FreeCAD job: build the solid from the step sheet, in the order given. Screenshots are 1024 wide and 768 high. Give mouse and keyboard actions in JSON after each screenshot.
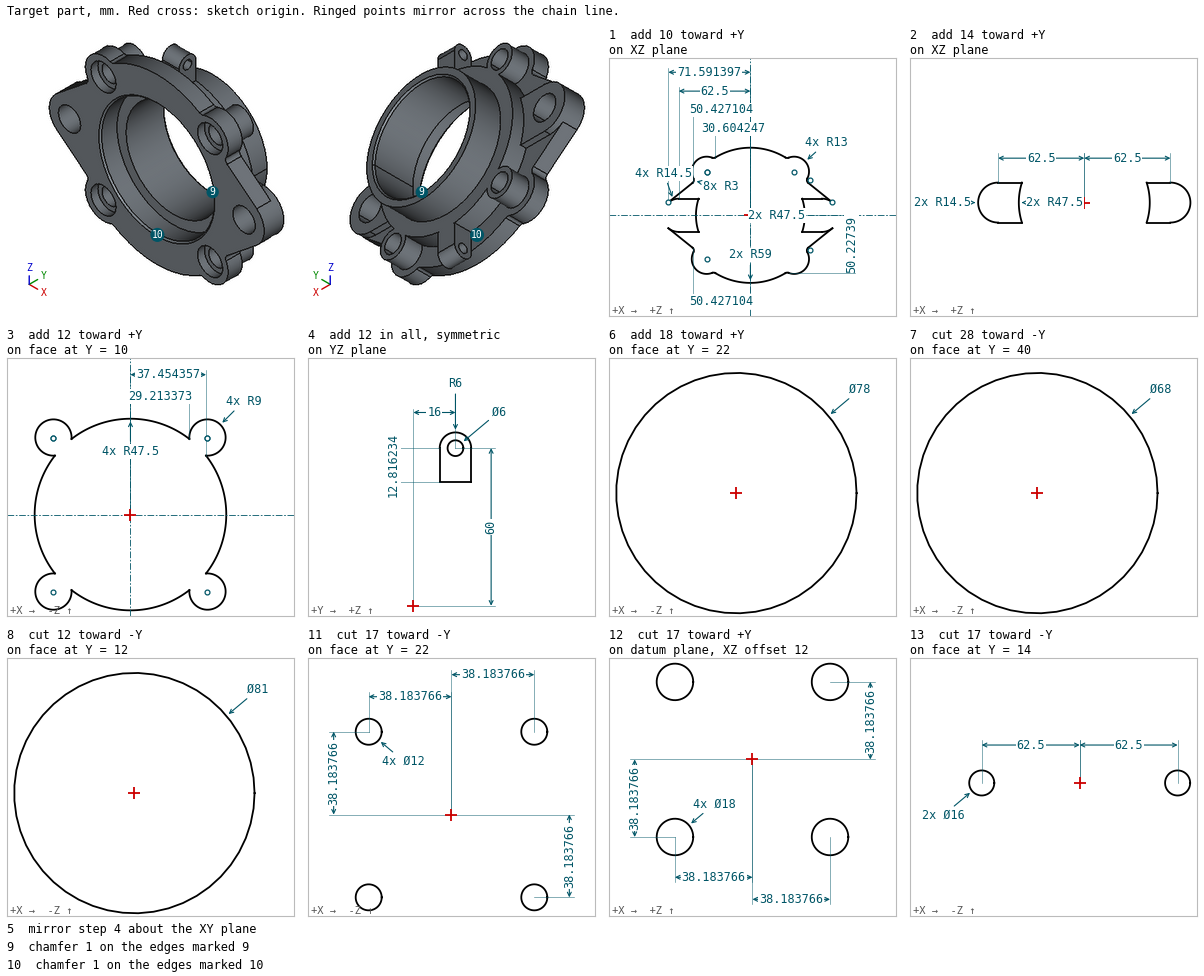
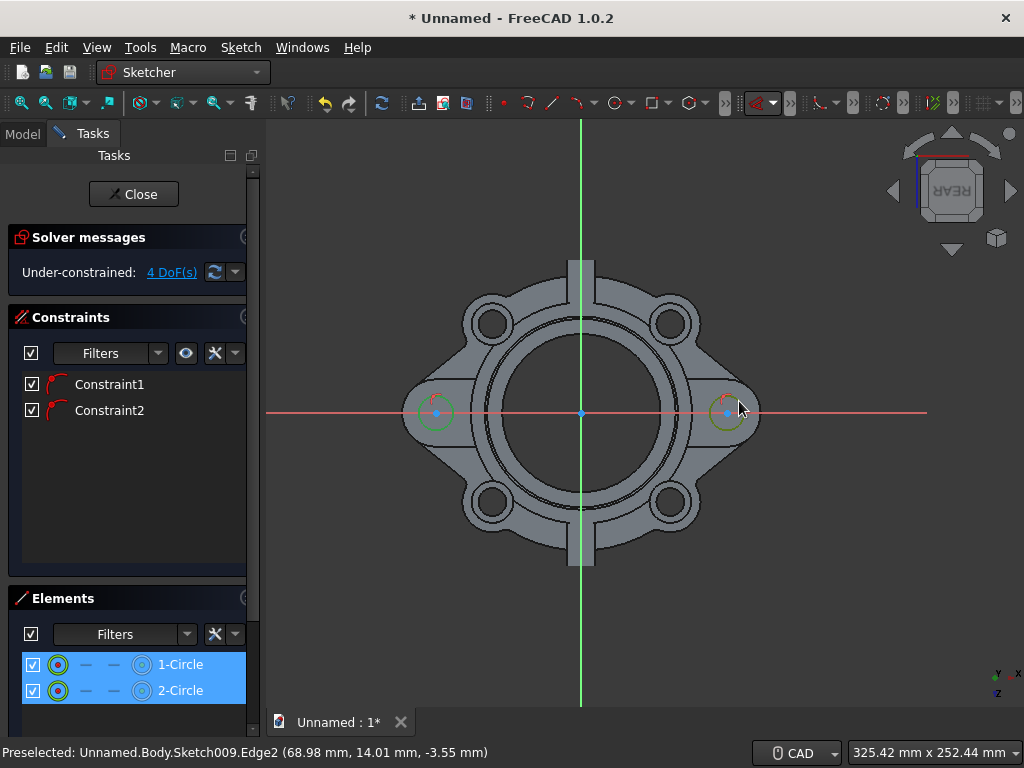
{"action": "key", "text": "e"}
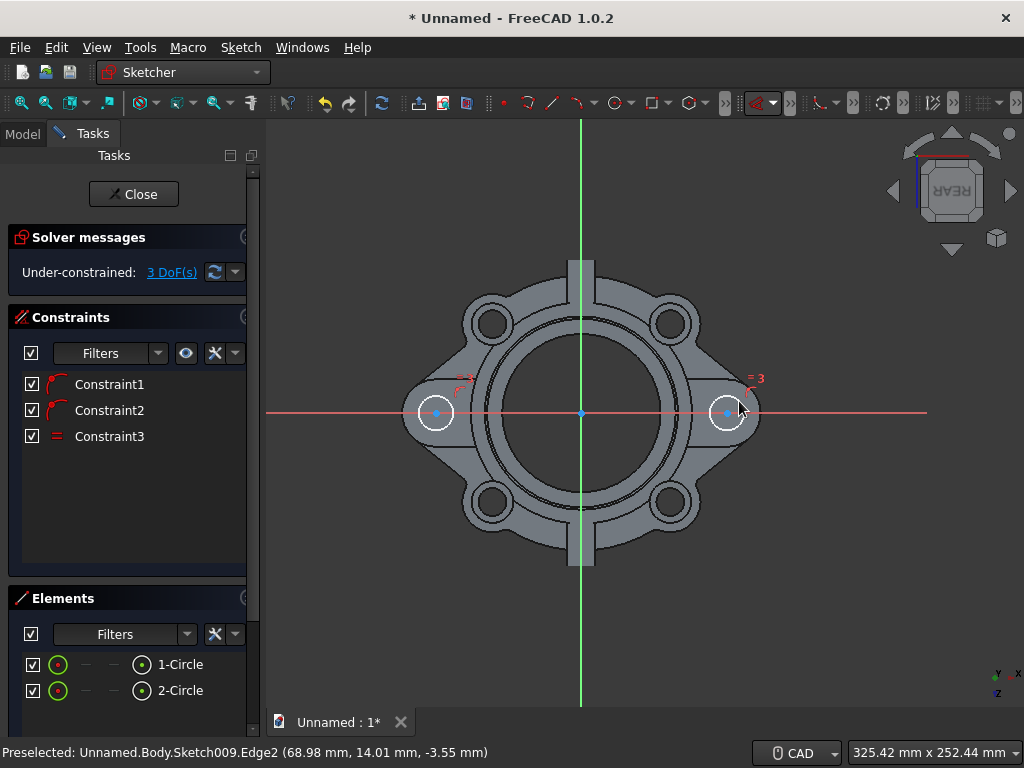
{"action": "key", "text": "d"}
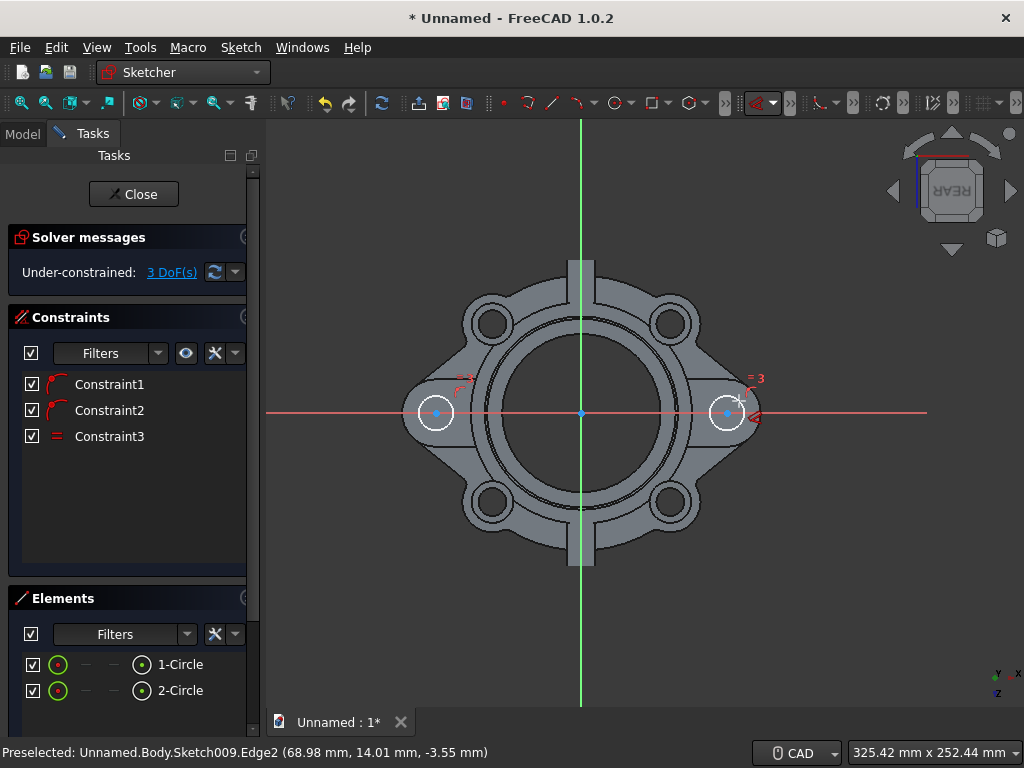
{"action": "left_click", "coordinate": [448, 401]}
{"action": "left_click", "coordinate": [471, 378]}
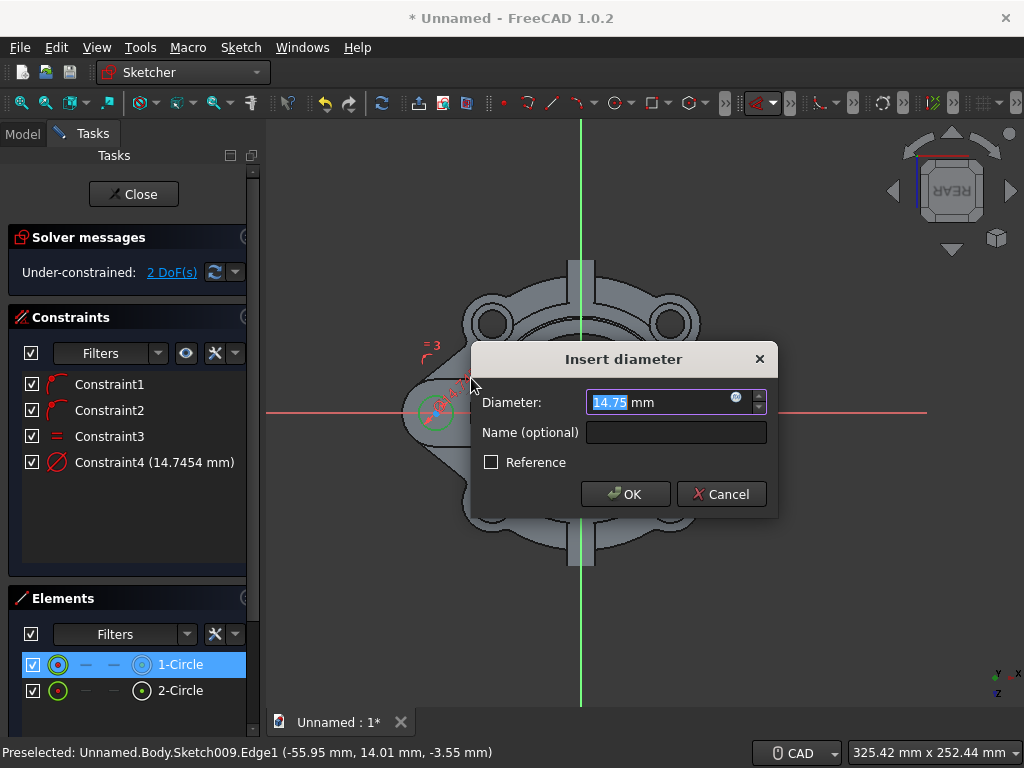
{"action": "type", "text": "16"}
{"action": "key", "text": "Return"}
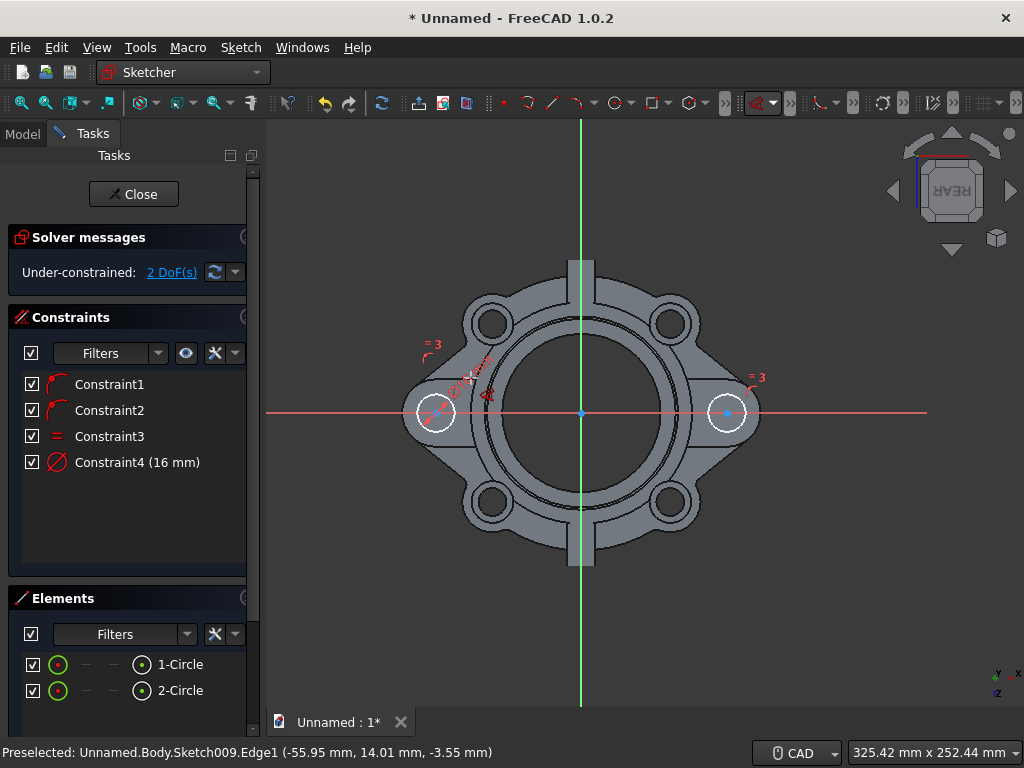
{"action": "left_click", "coordinate": [436, 413]}
{"action": "left_click", "coordinate": [509, 447]}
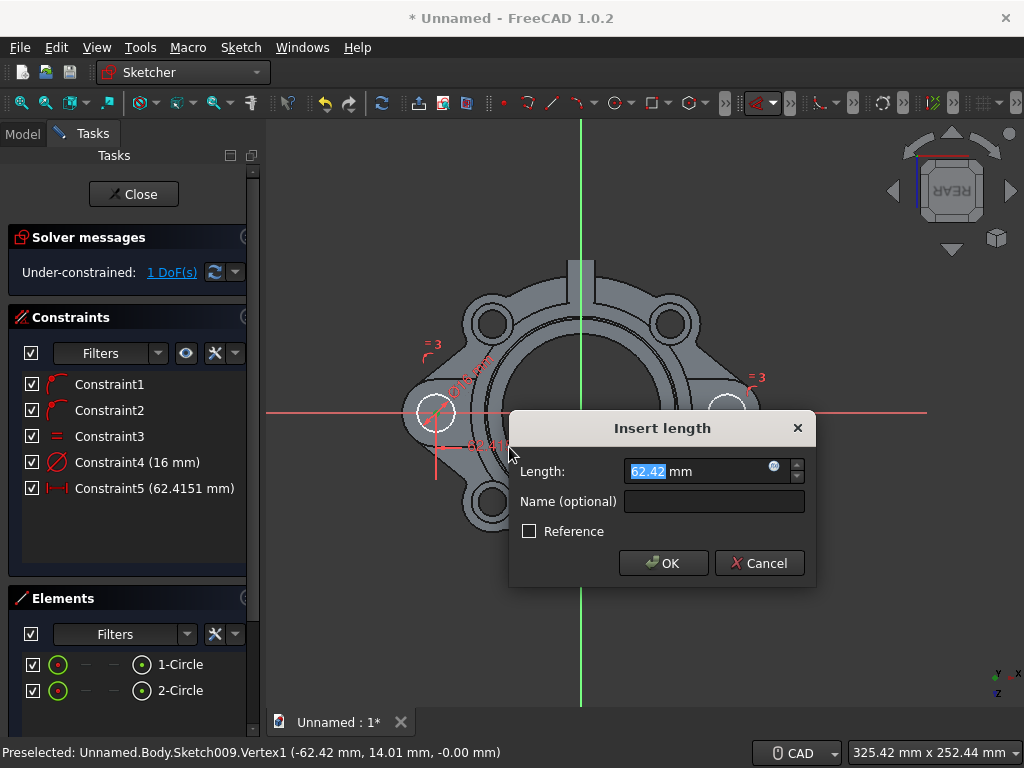
{"action": "type", "text": "62.5"}
{"action": "key", "text": "Return"}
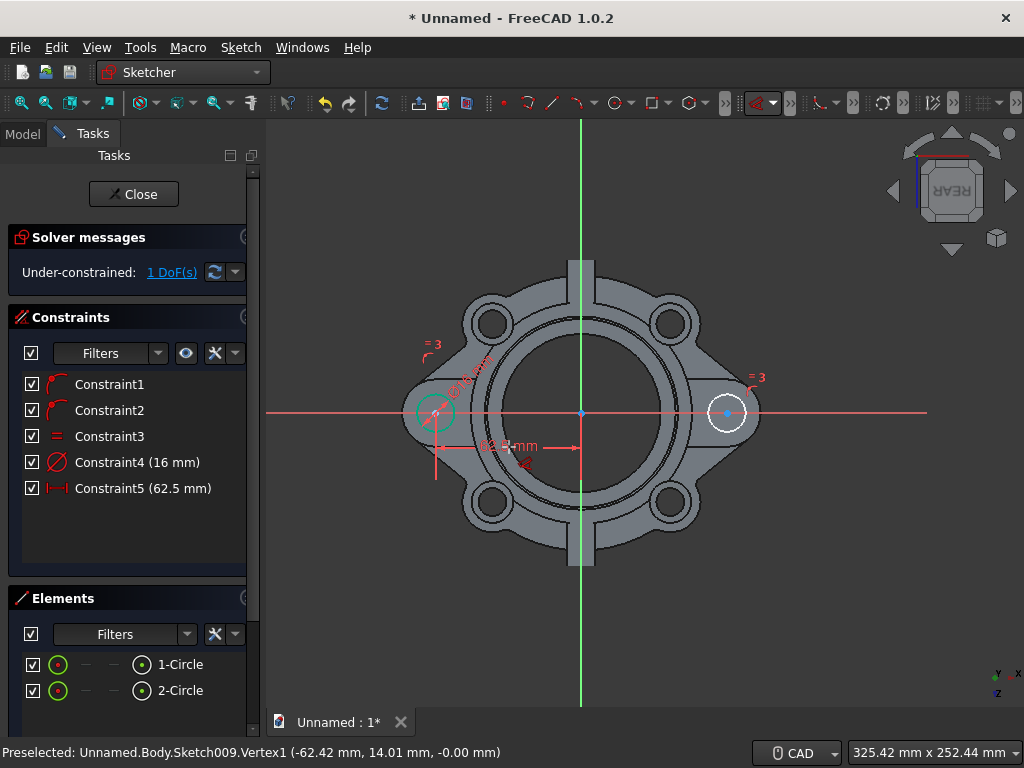
{"action": "left_click", "coordinate": [727, 413]}
{"action": "left_click", "coordinate": [654, 447]}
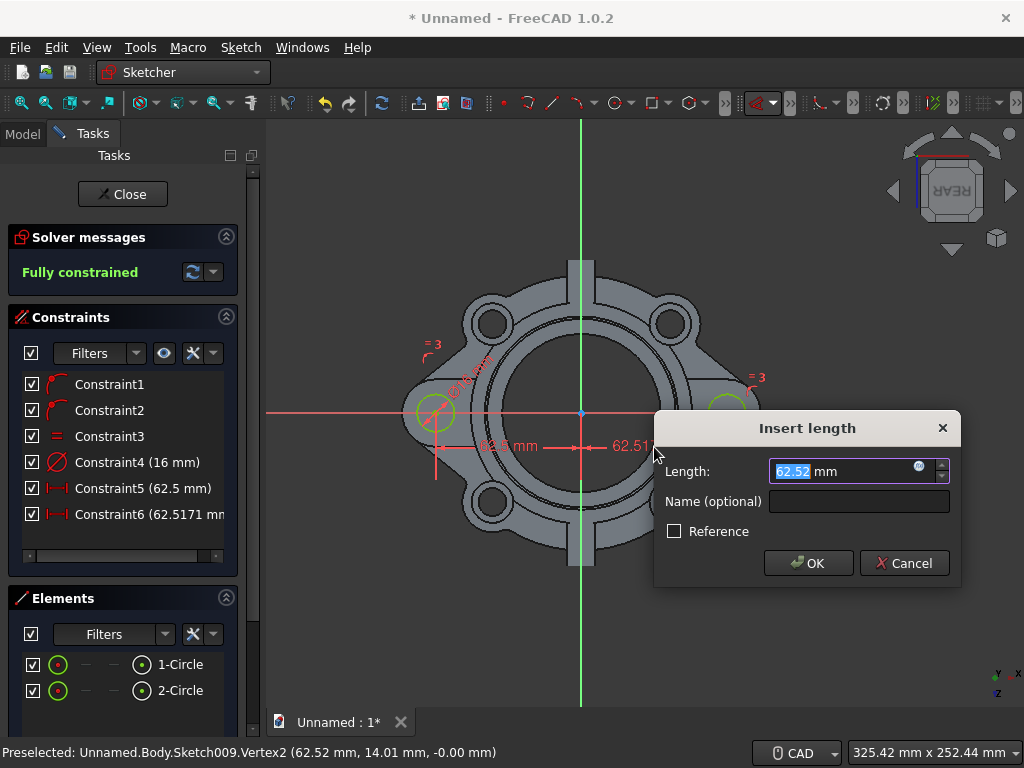
{"action": "type", "text": "62.5"}
{"action": "key", "text": "Return"}
{"action": "key", "text": "Escape"}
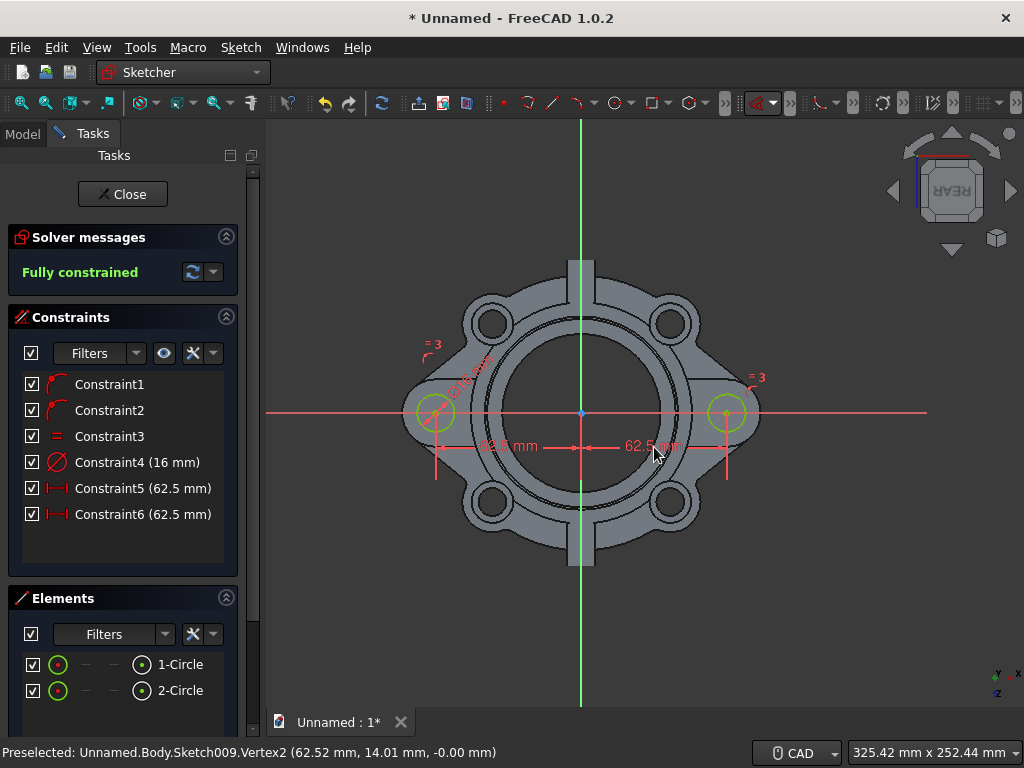
{"action": "left_click", "coordinate": [123, 194]}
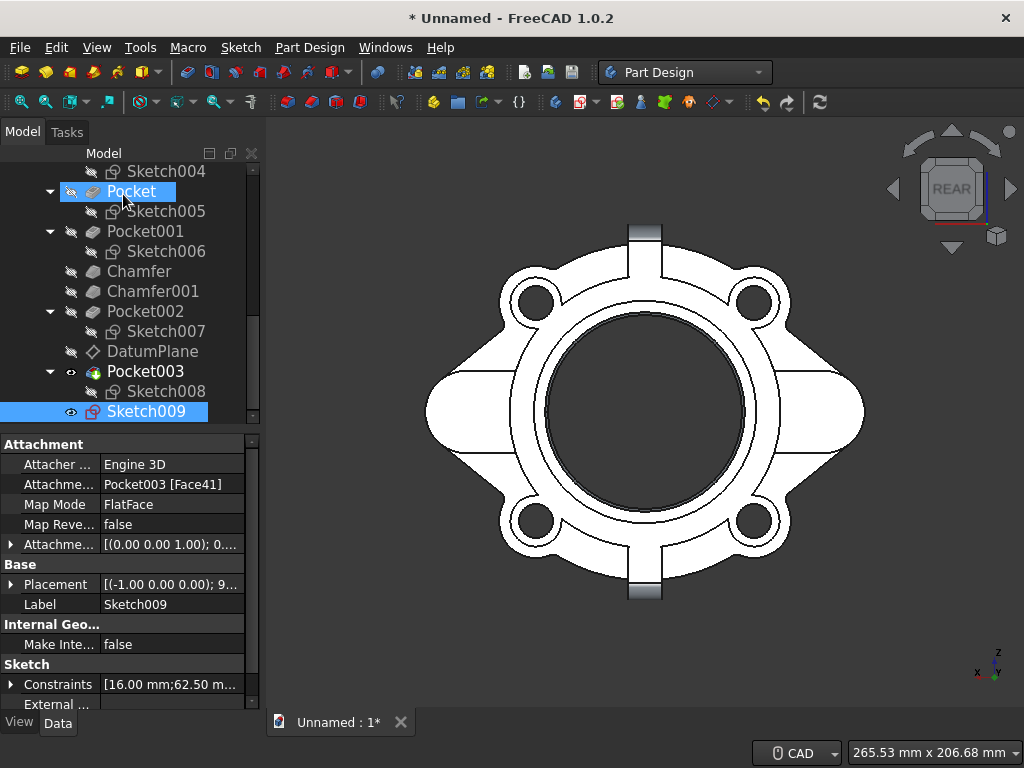
{"action": "left_click", "coordinate": [188, 72]}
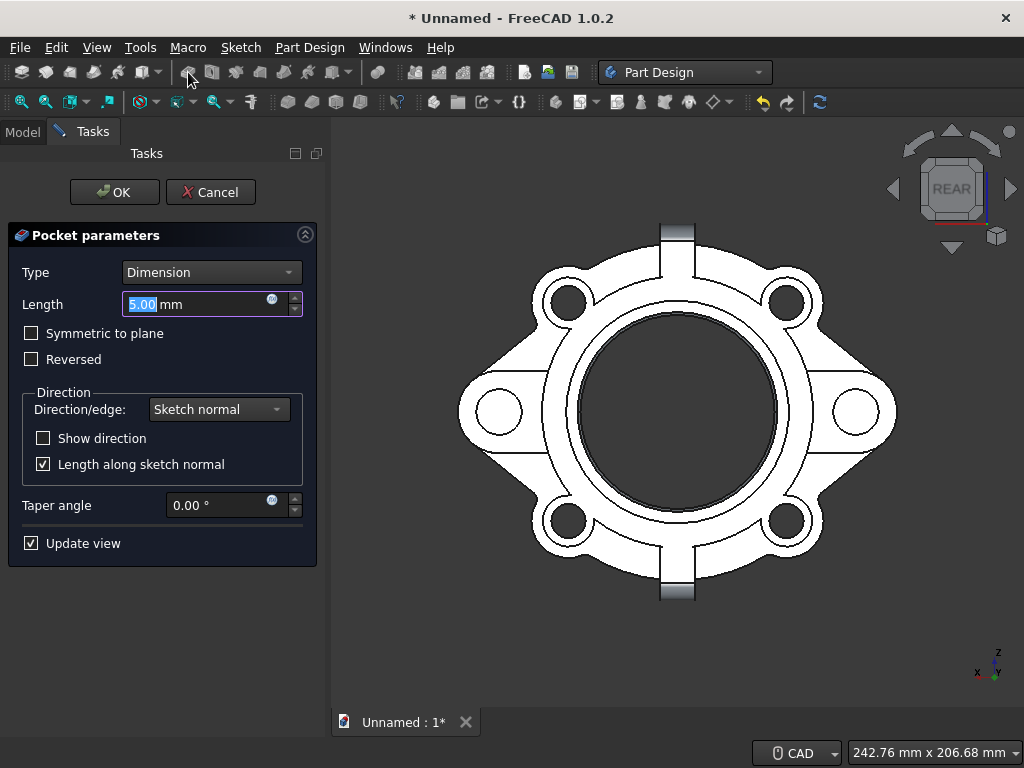
{"action": "type", "text": "17"}
{"action": "key", "text": "Tab"}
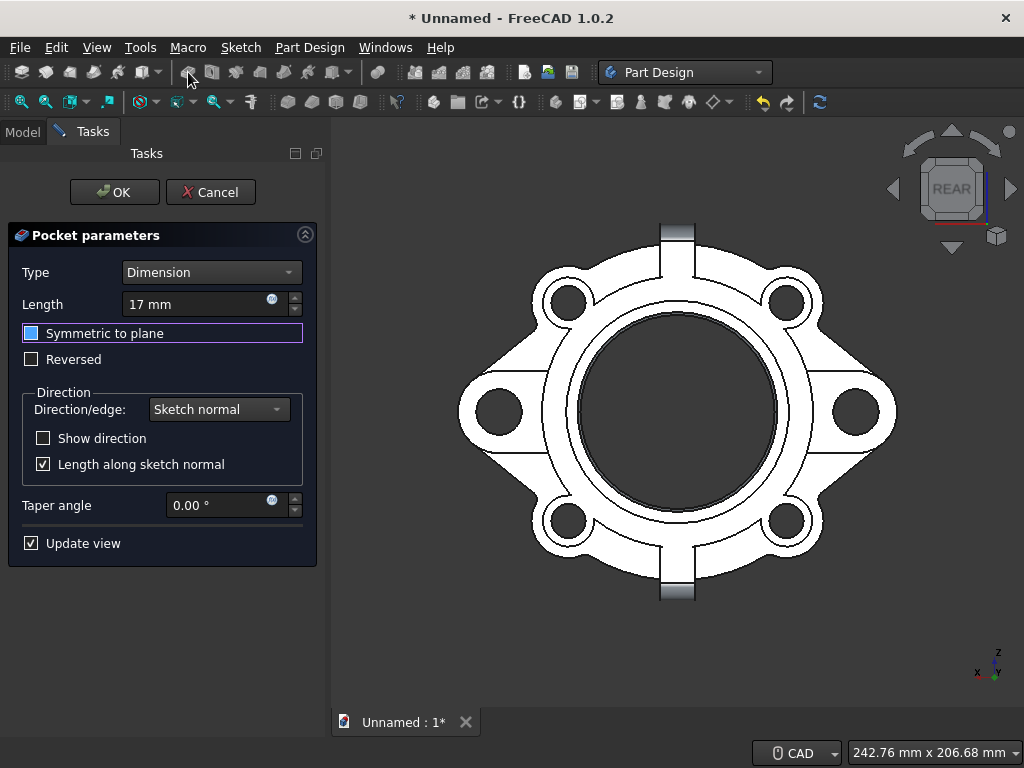
{"action": "left_click", "coordinate": [115, 192]}